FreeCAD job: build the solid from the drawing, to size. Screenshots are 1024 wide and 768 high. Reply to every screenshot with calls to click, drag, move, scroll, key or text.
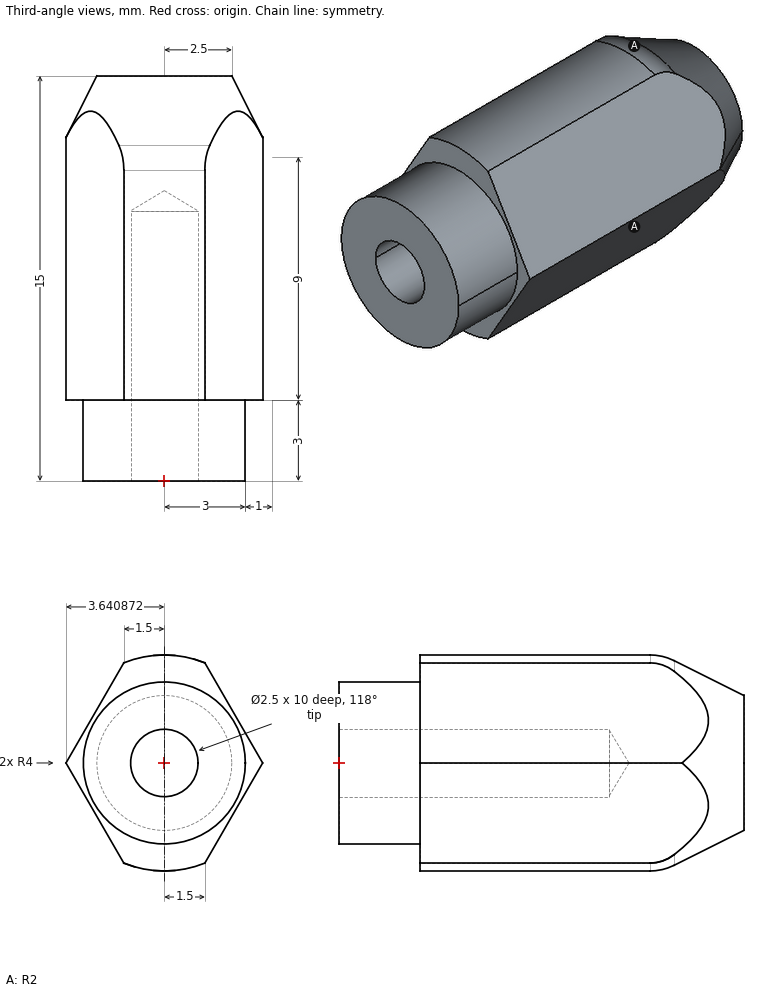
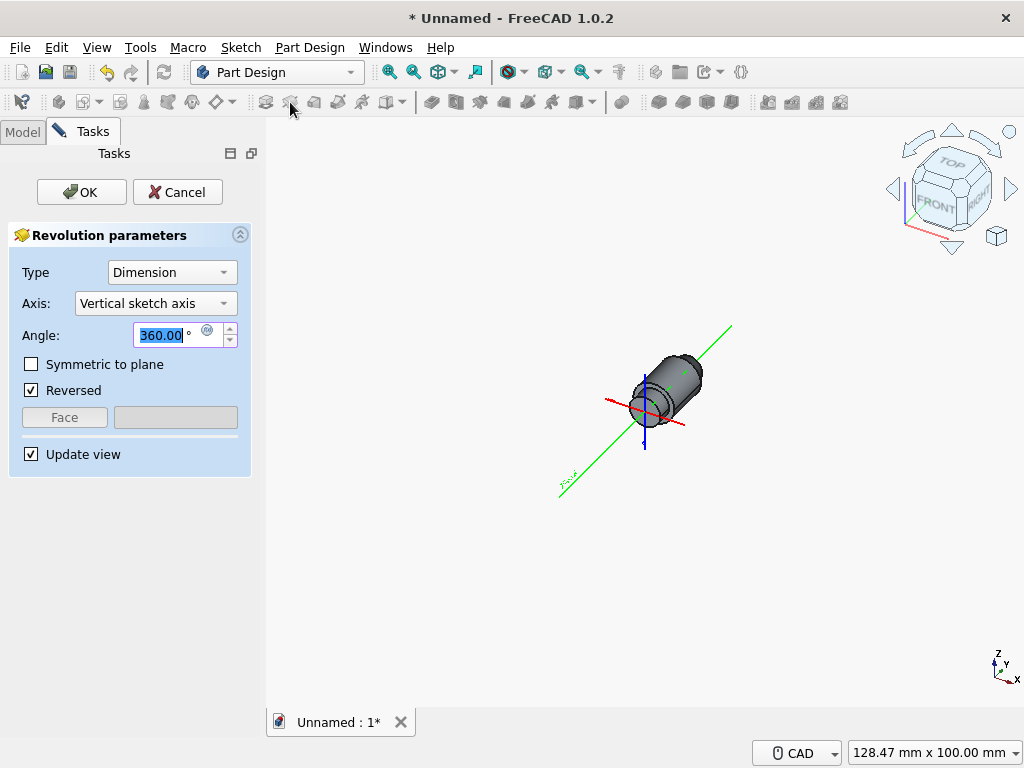
click(82, 192)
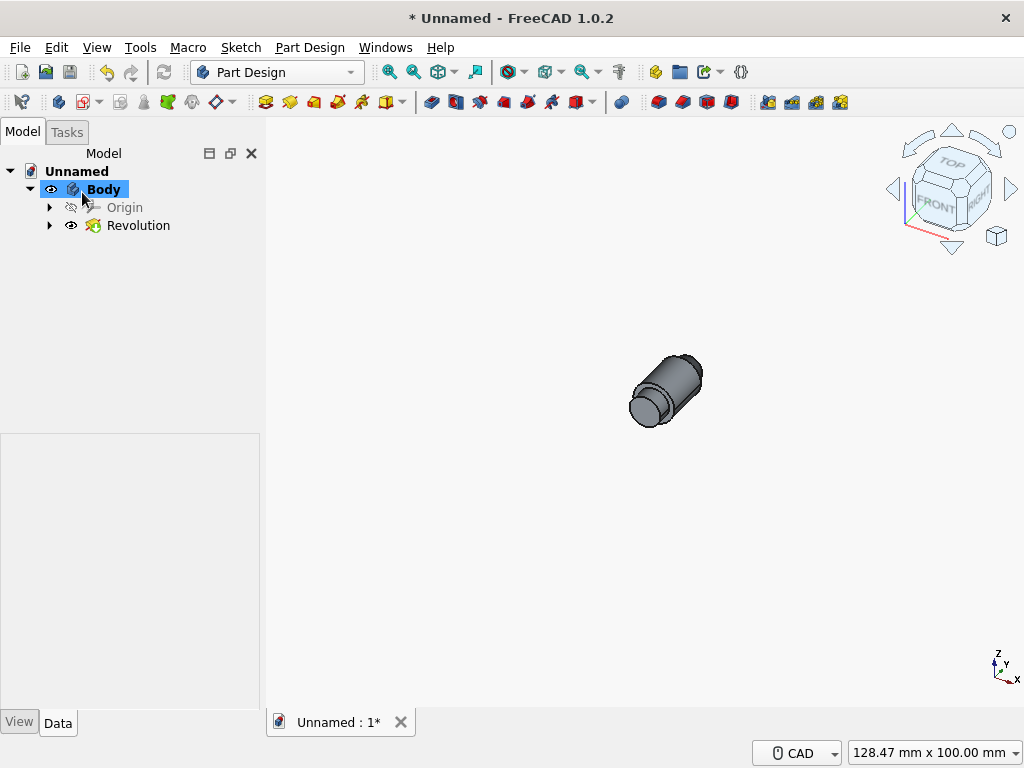
click(390, 72)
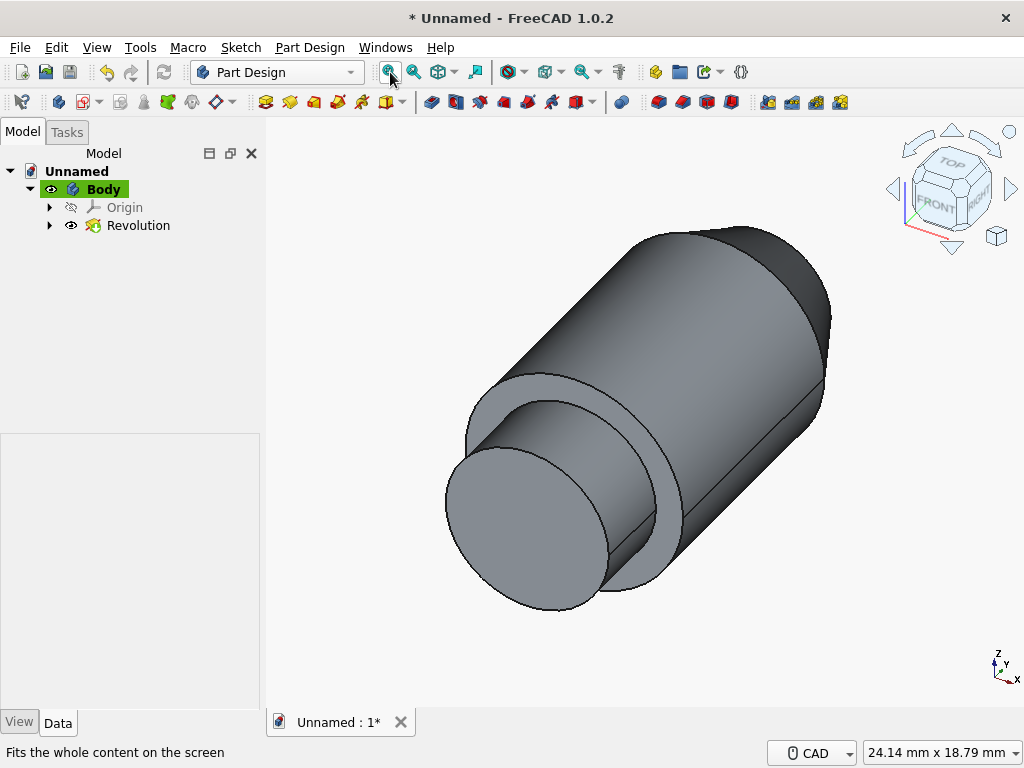
click(527, 528)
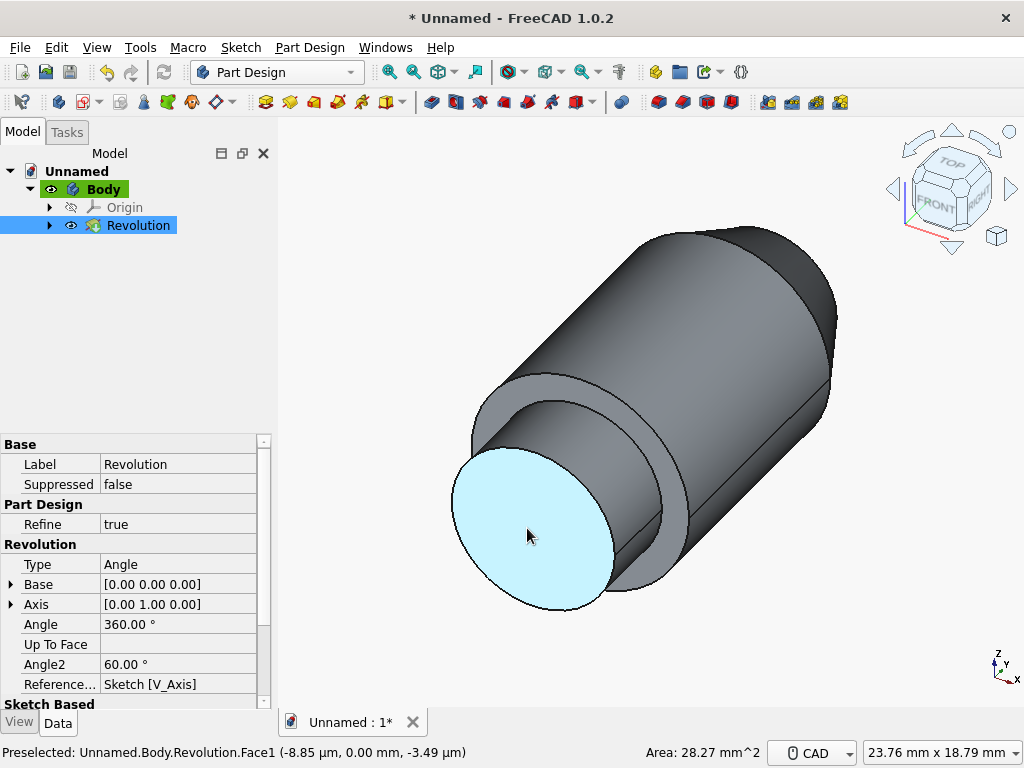
click(84, 102)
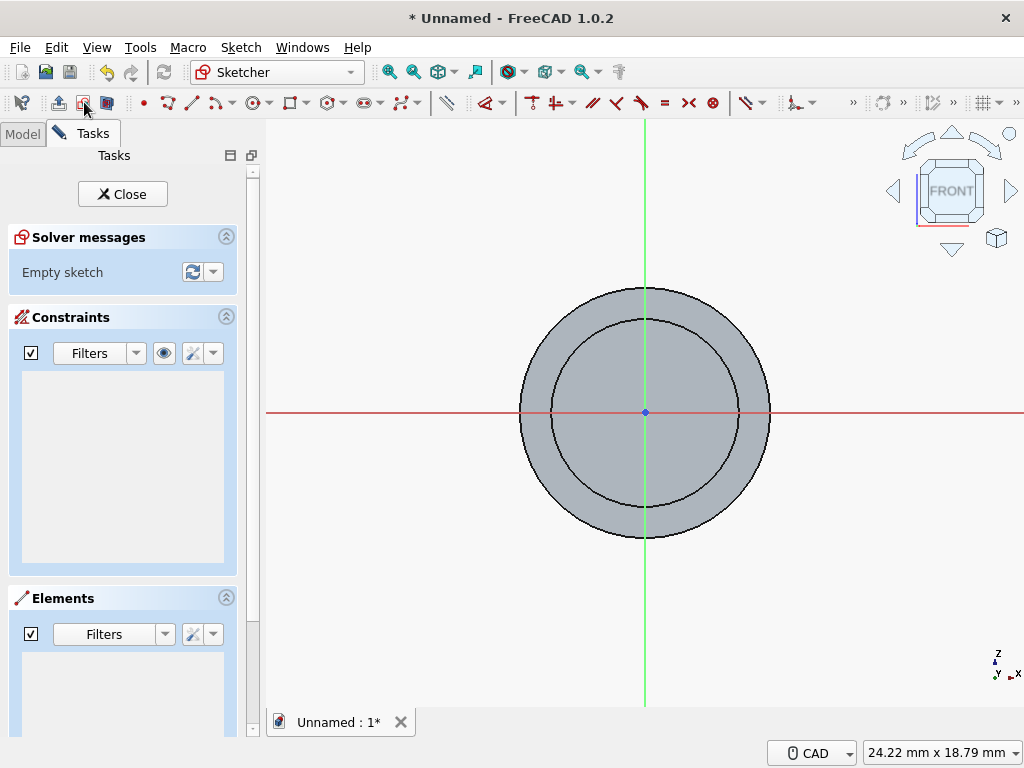
scroll(662, 413, up, 8)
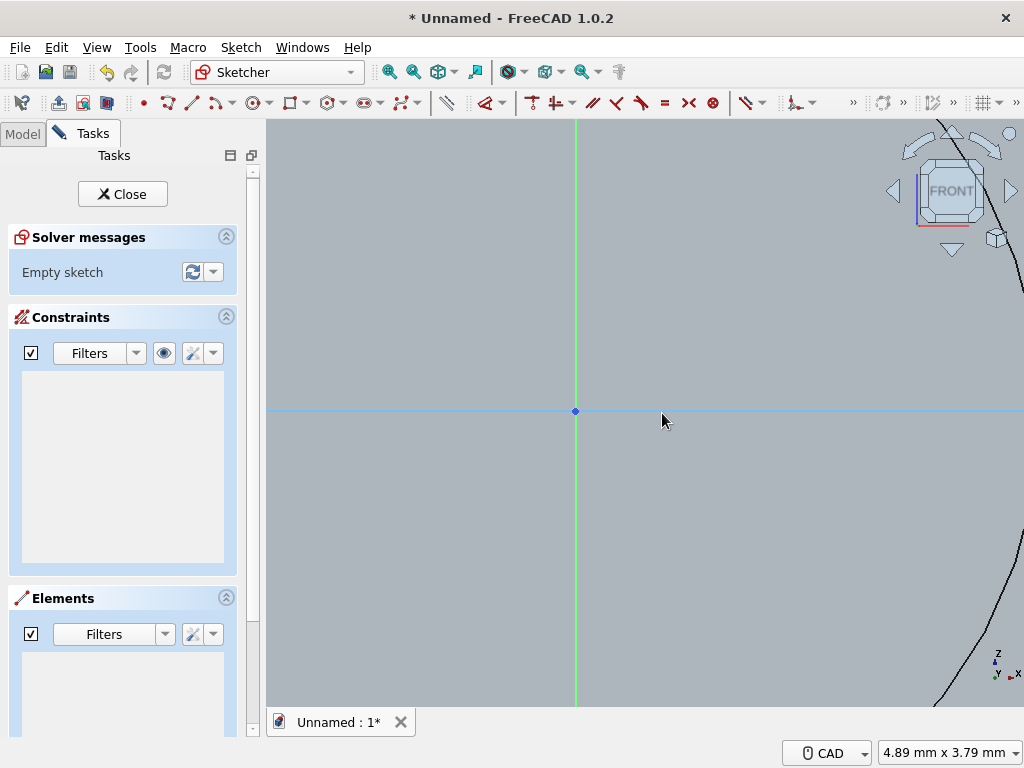
click(254, 104)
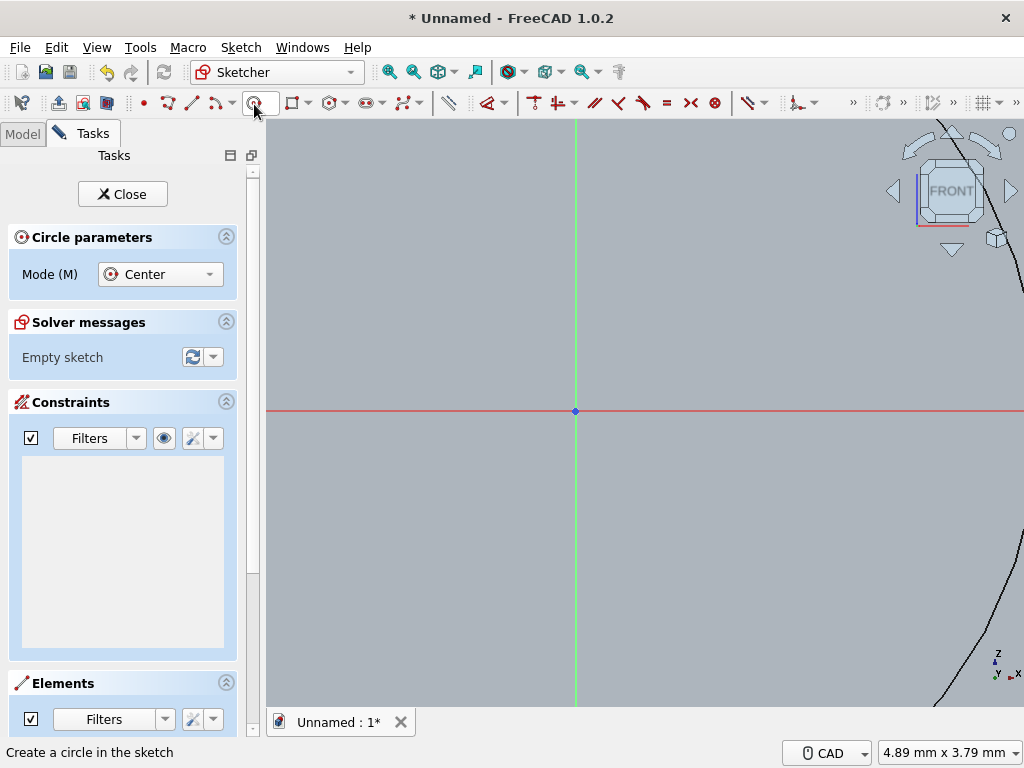
click(576, 411)
click(713, 274)
key(Escape)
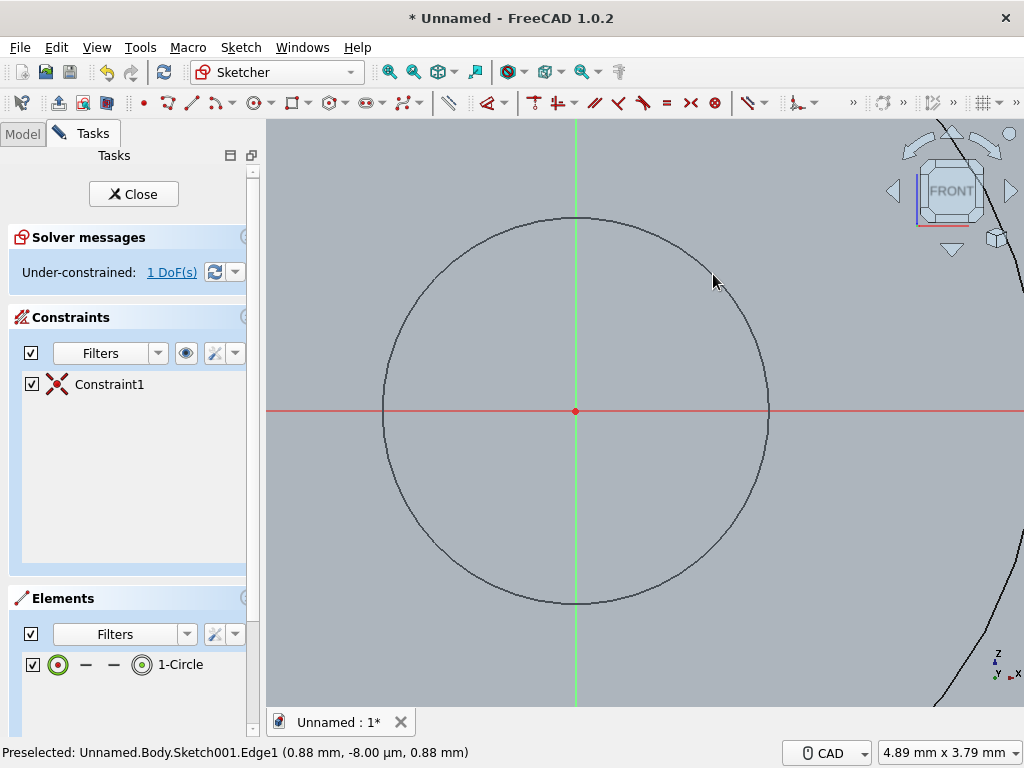
click(488, 104)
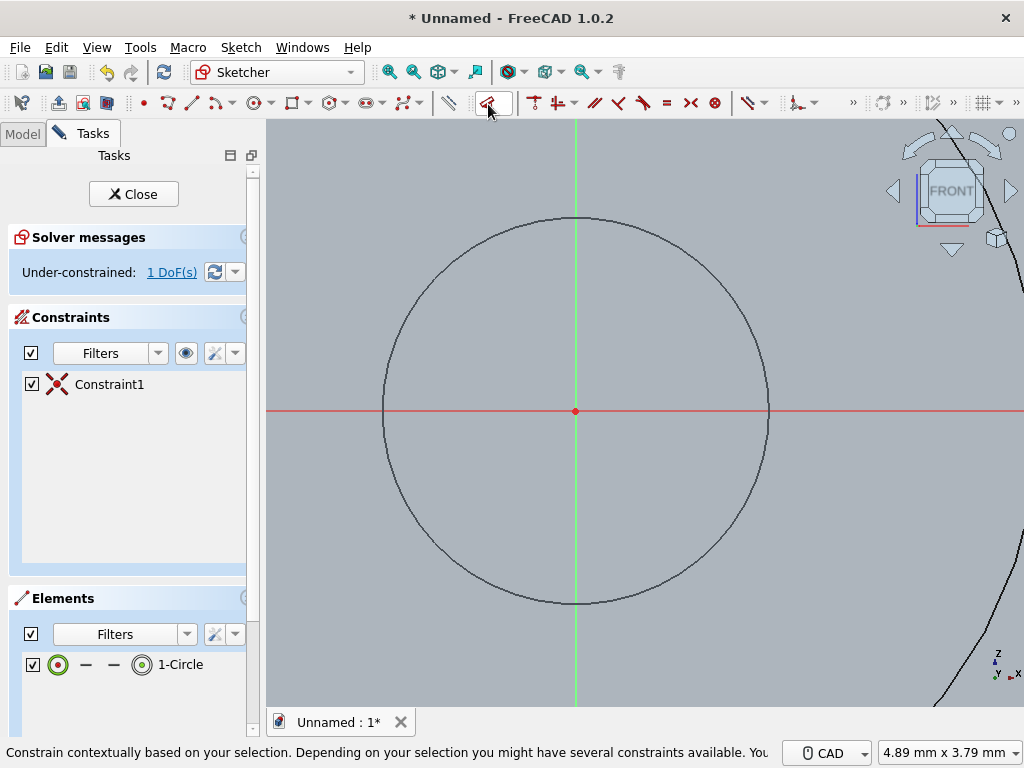
click(712, 274)
click(735, 251)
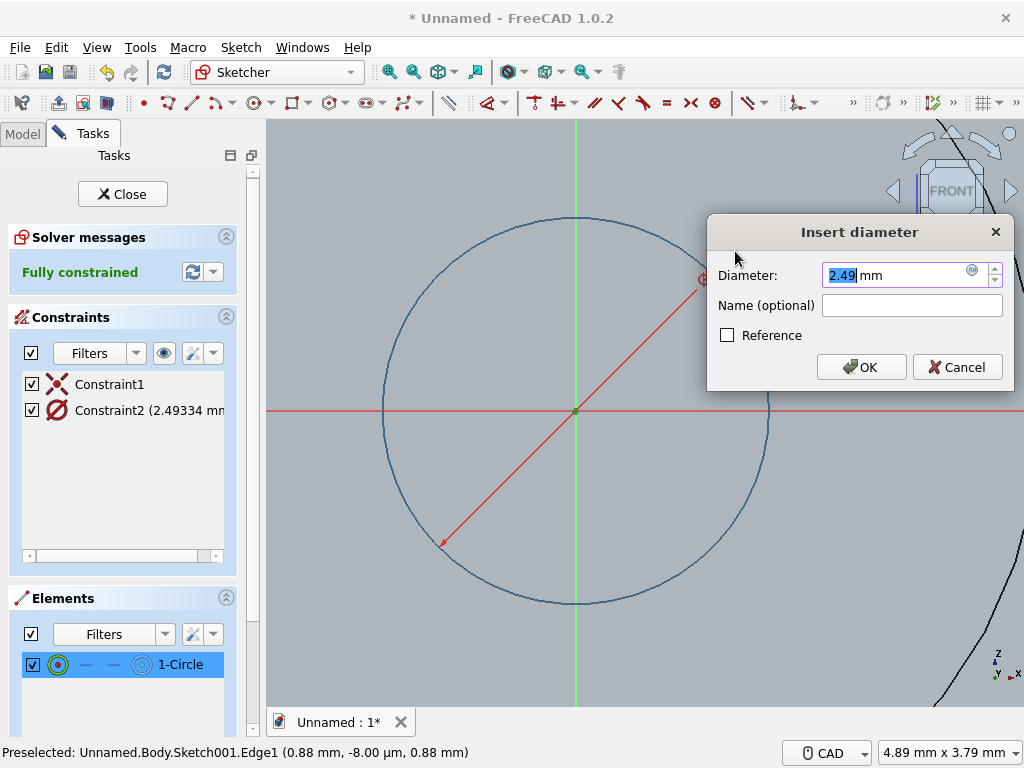
text(2.5)
key(Return)
key(Escape)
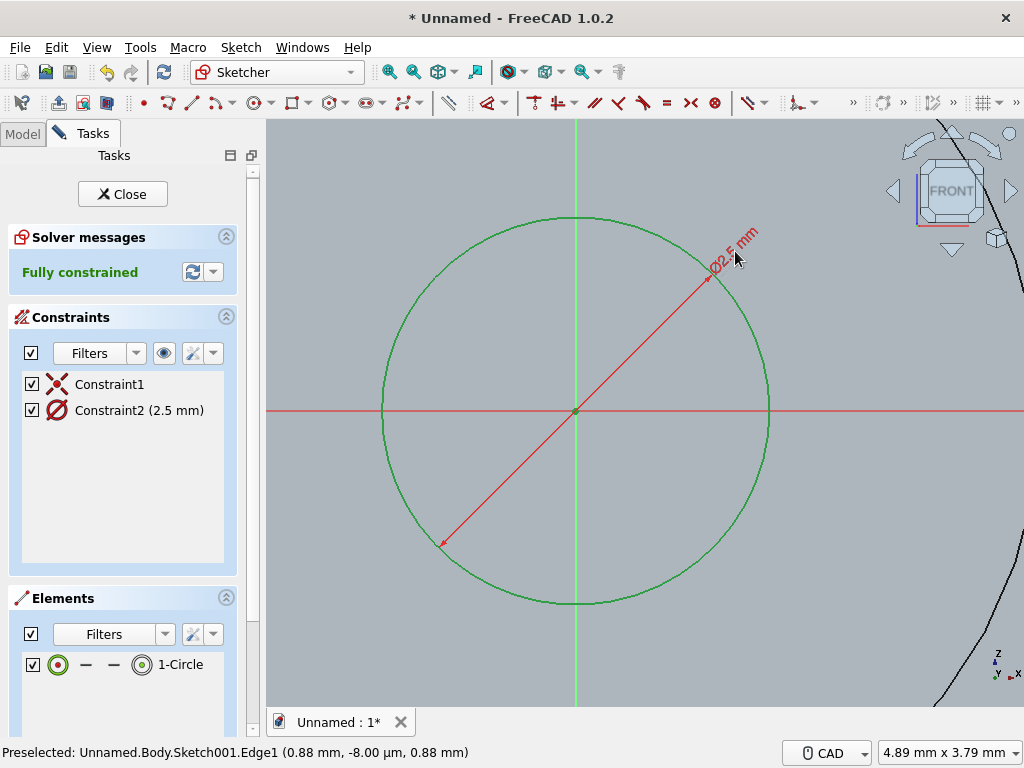
click(123, 194)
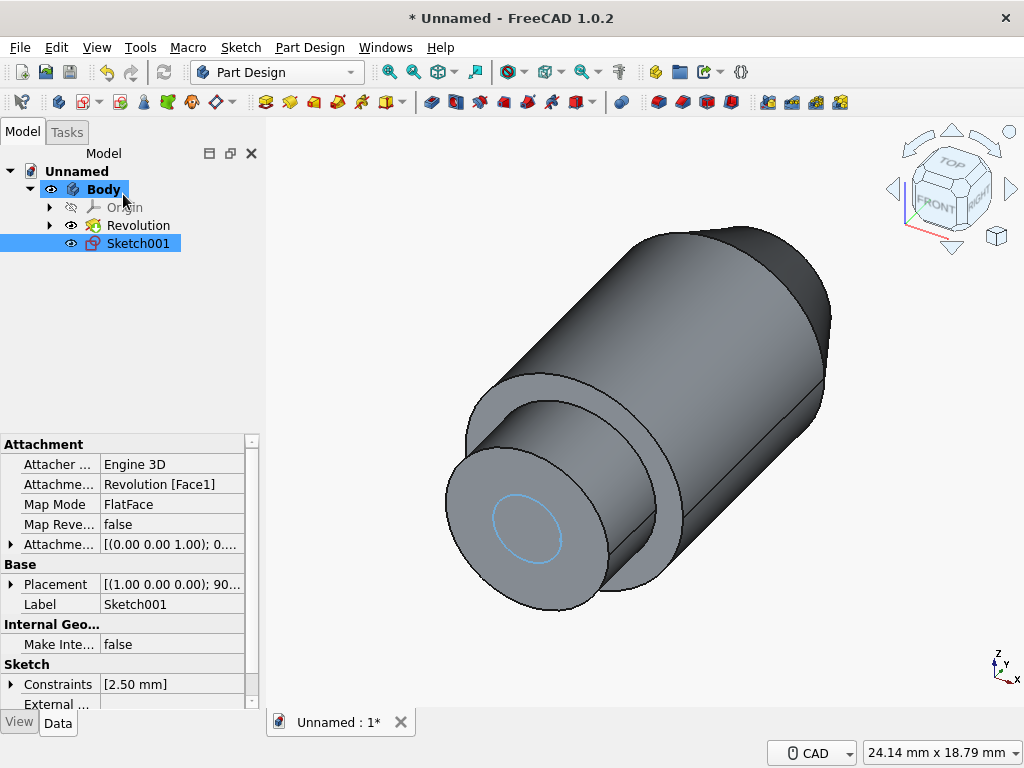
click(456, 102)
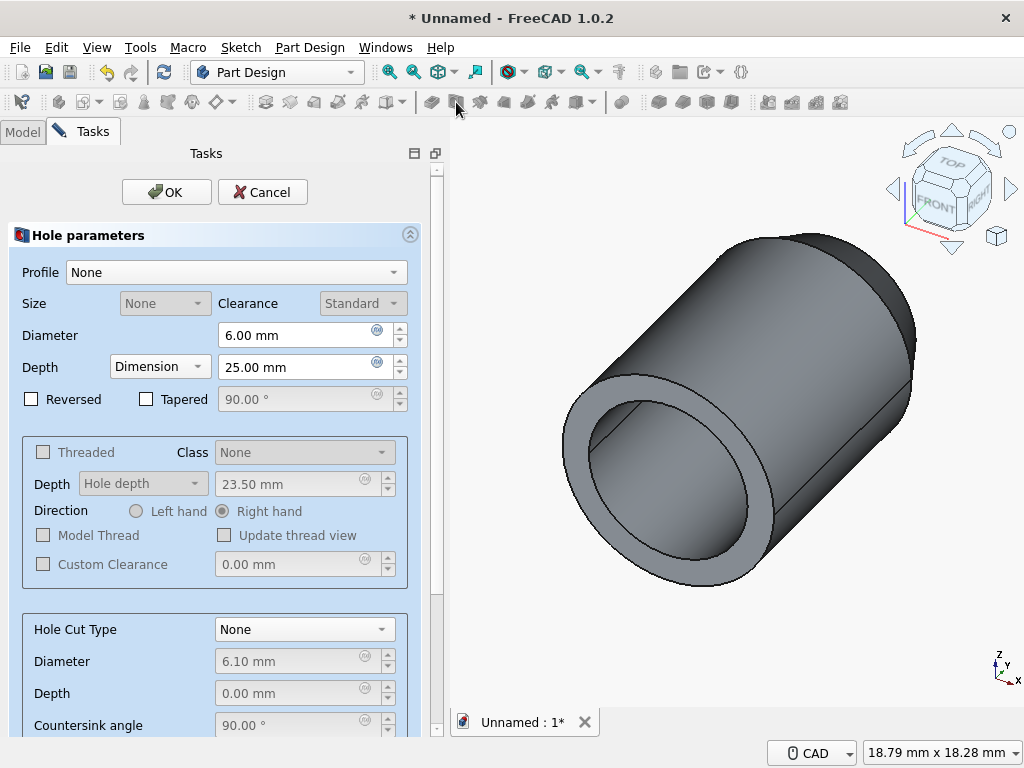
triple_click(305, 335)